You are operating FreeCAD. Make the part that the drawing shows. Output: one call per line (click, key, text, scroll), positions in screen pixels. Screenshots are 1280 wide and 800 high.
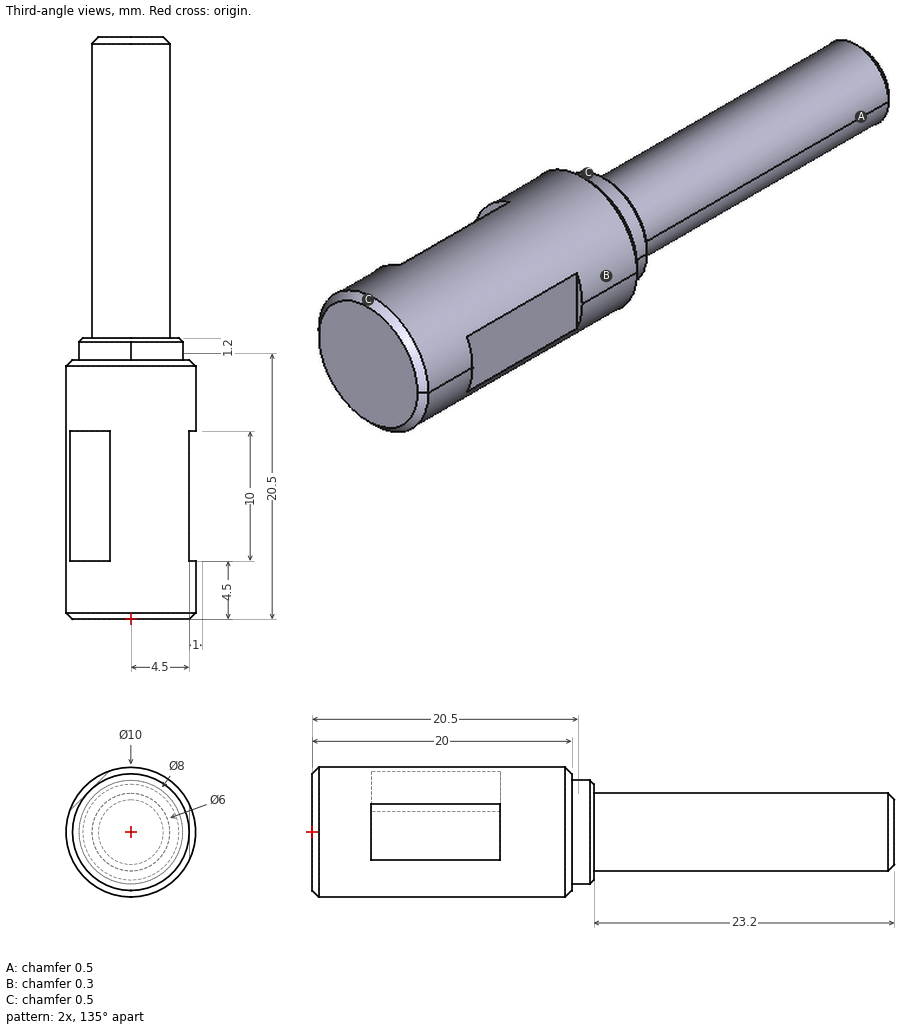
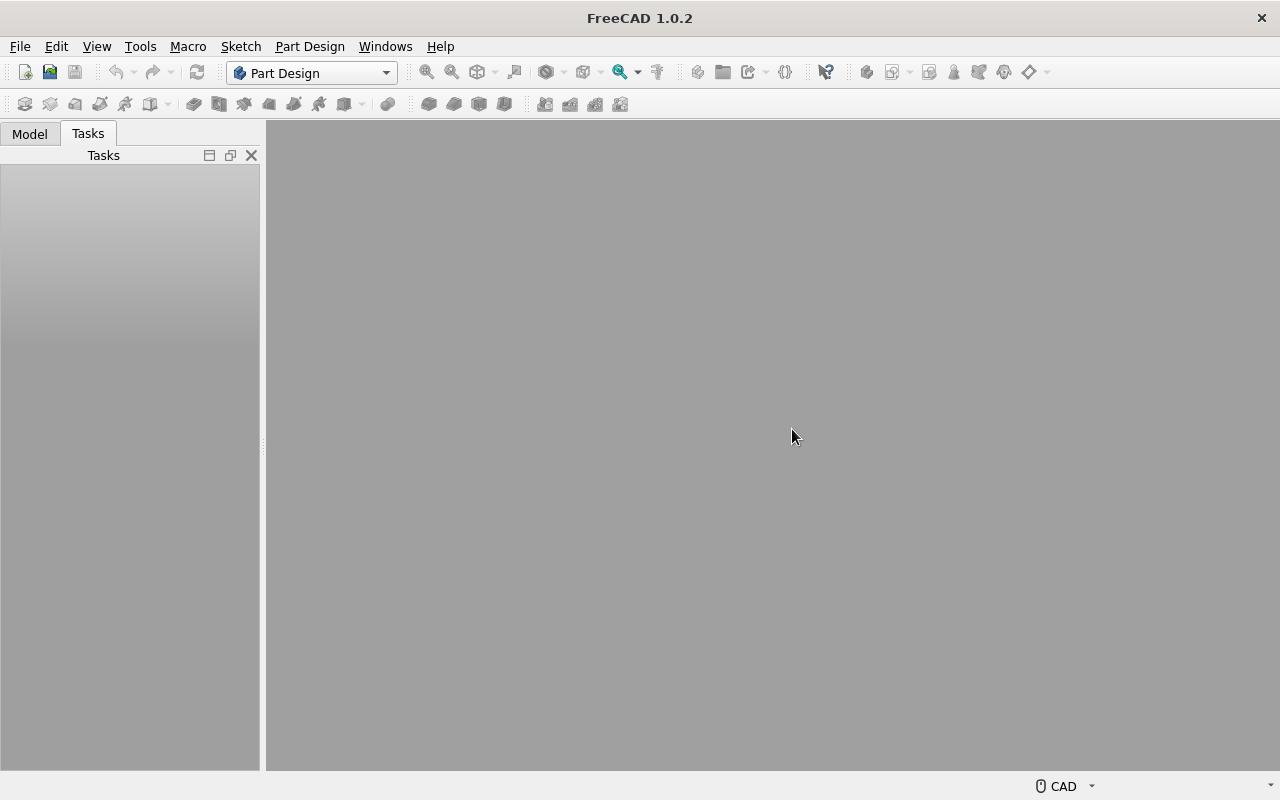
click(25, 72)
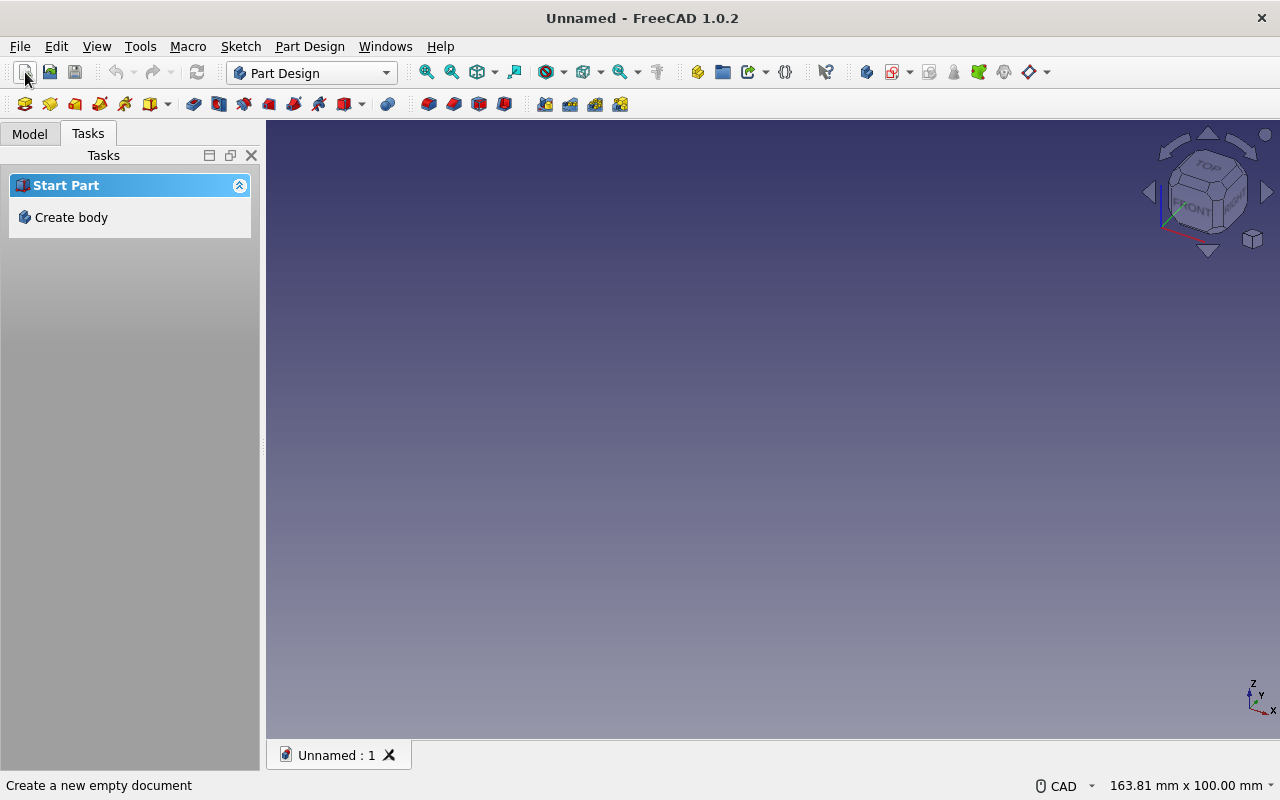
click(892, 72)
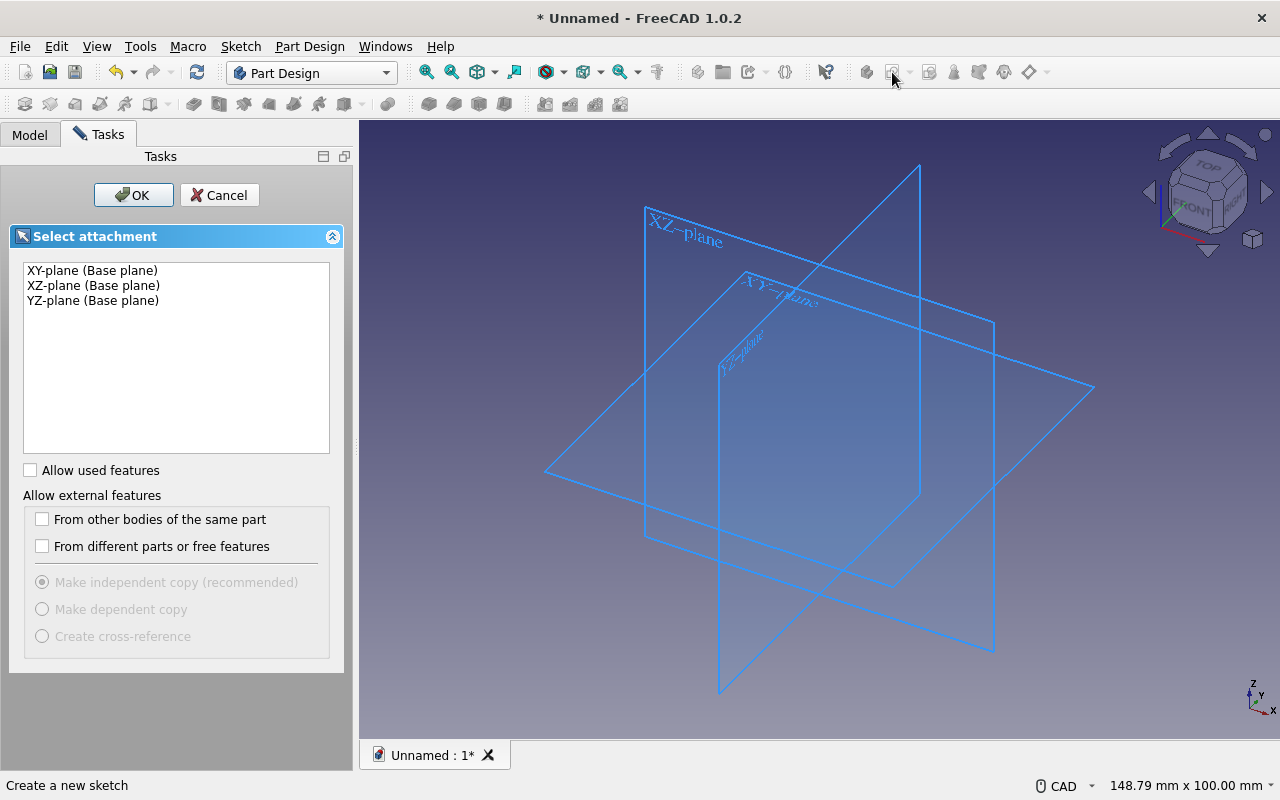
click(84, 286)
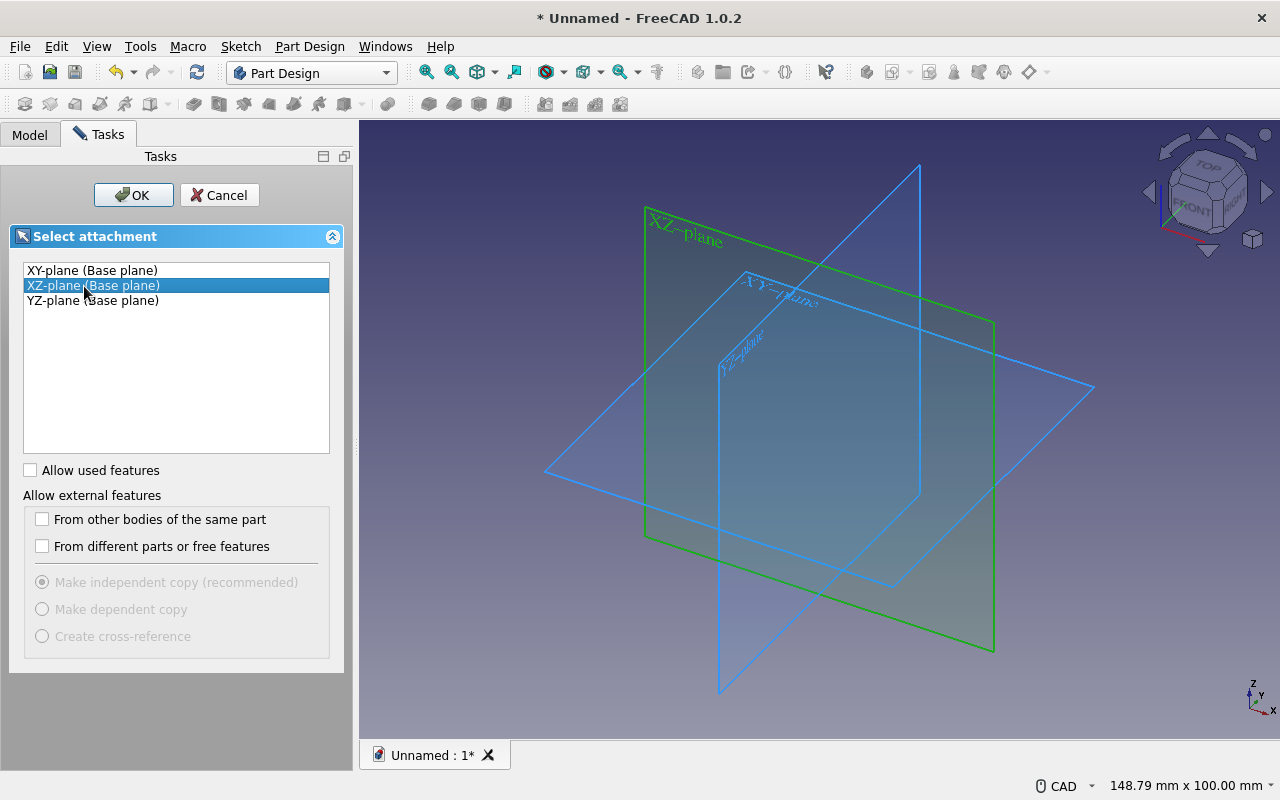
click(134, 195)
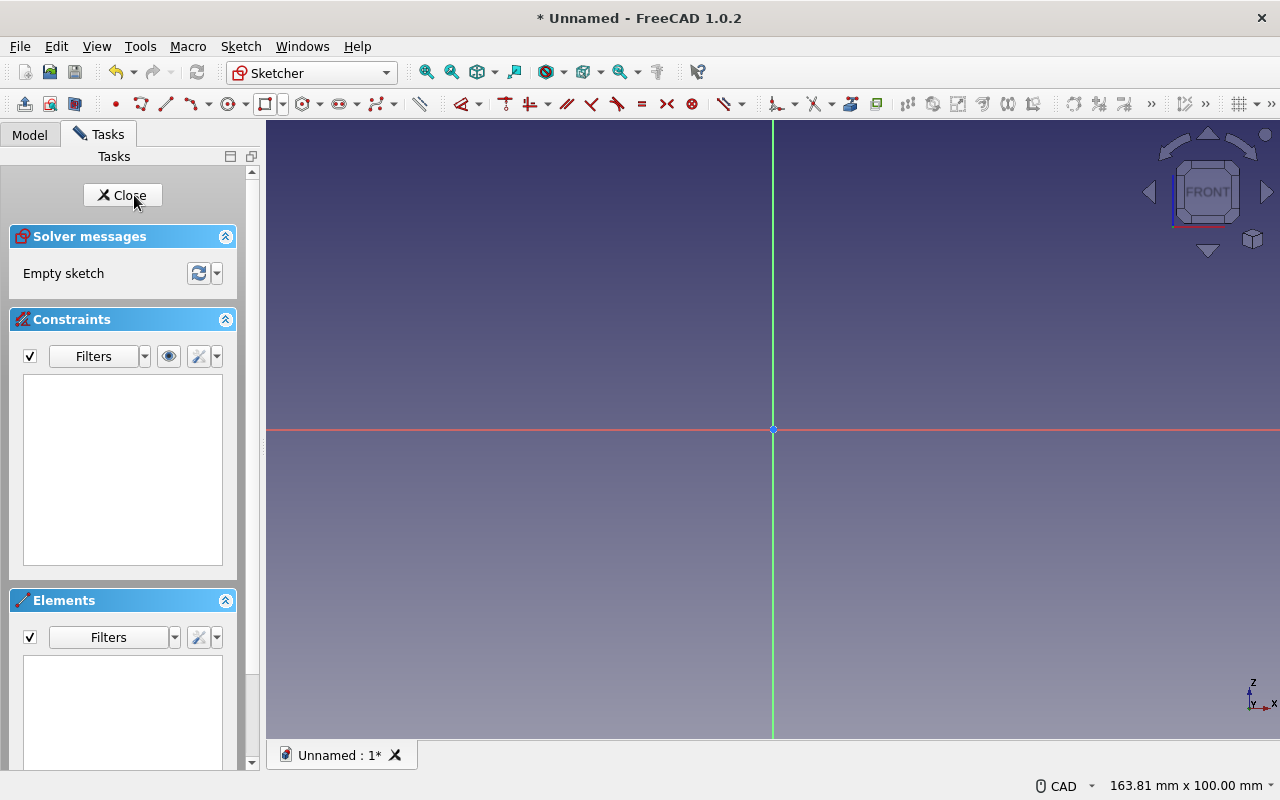
scroll(780, 429, up, 12)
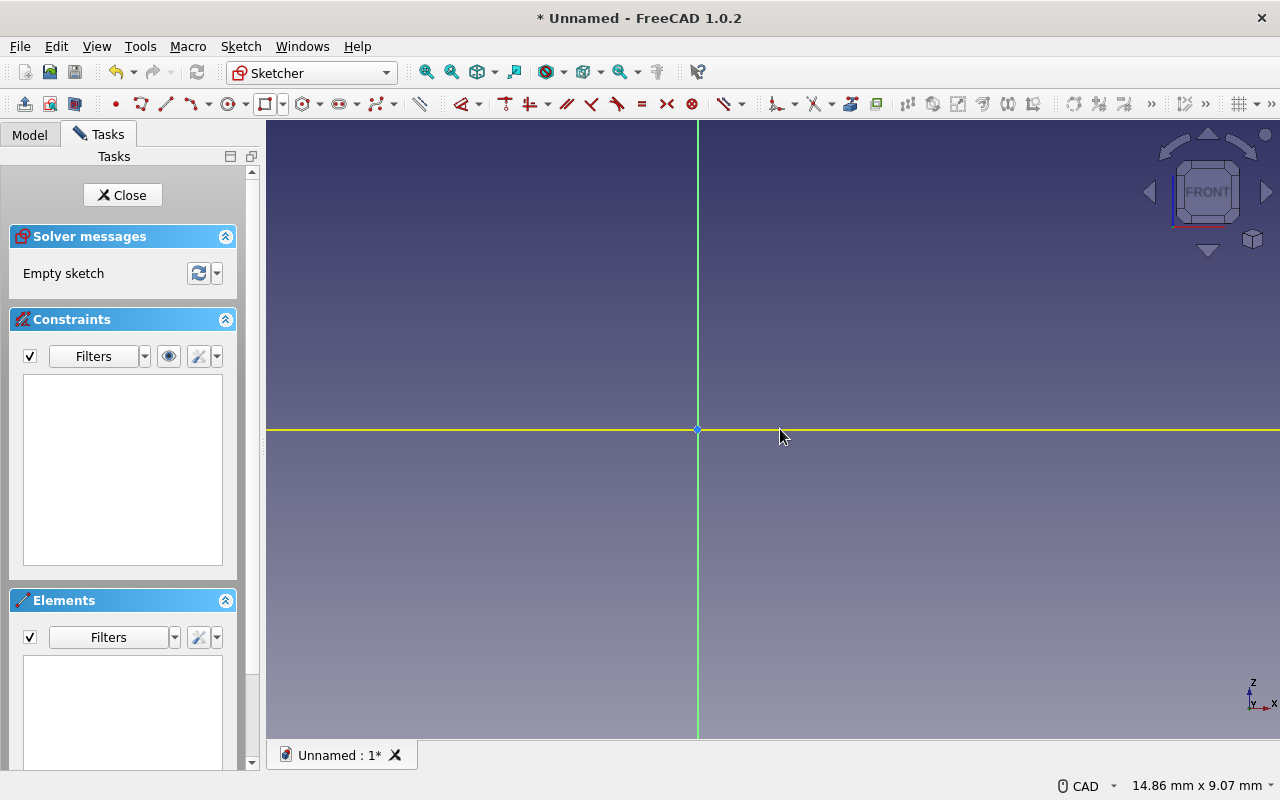
click(228, 104)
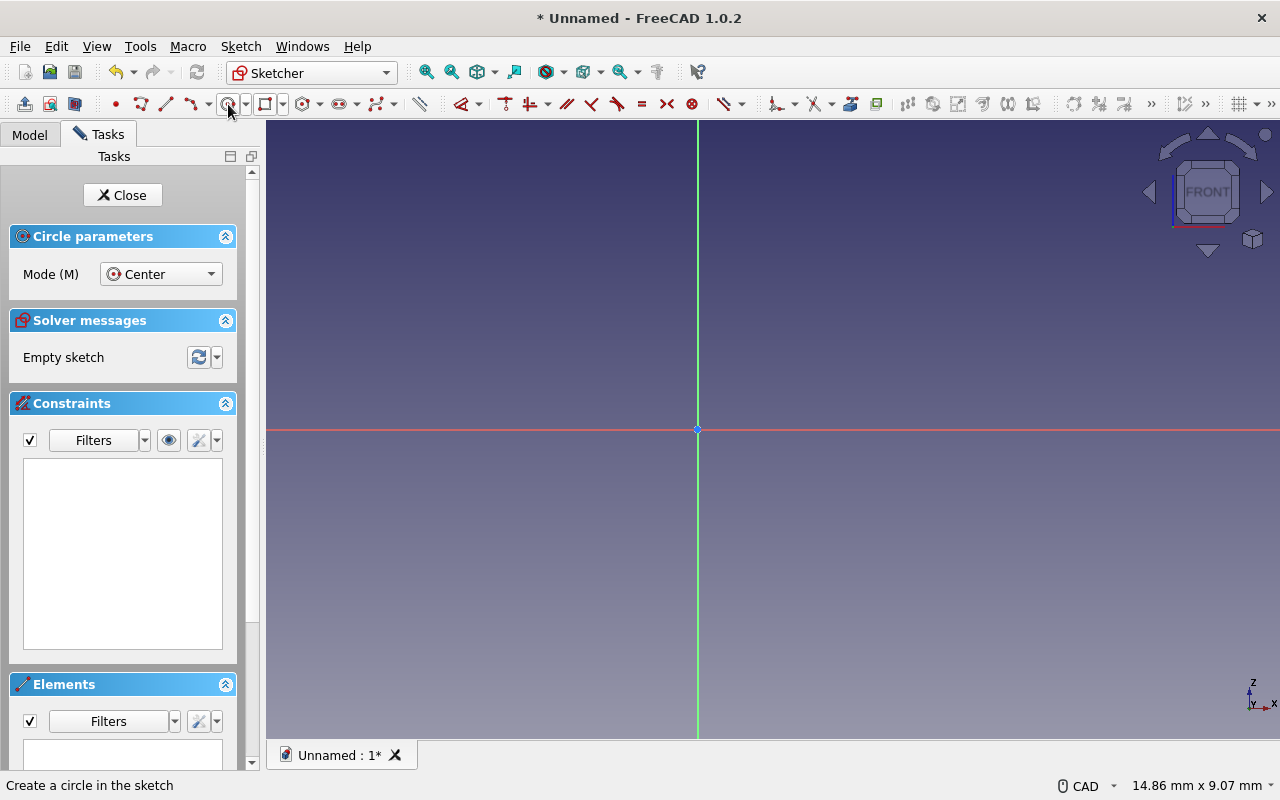
click(698, 430)
move(842, 285)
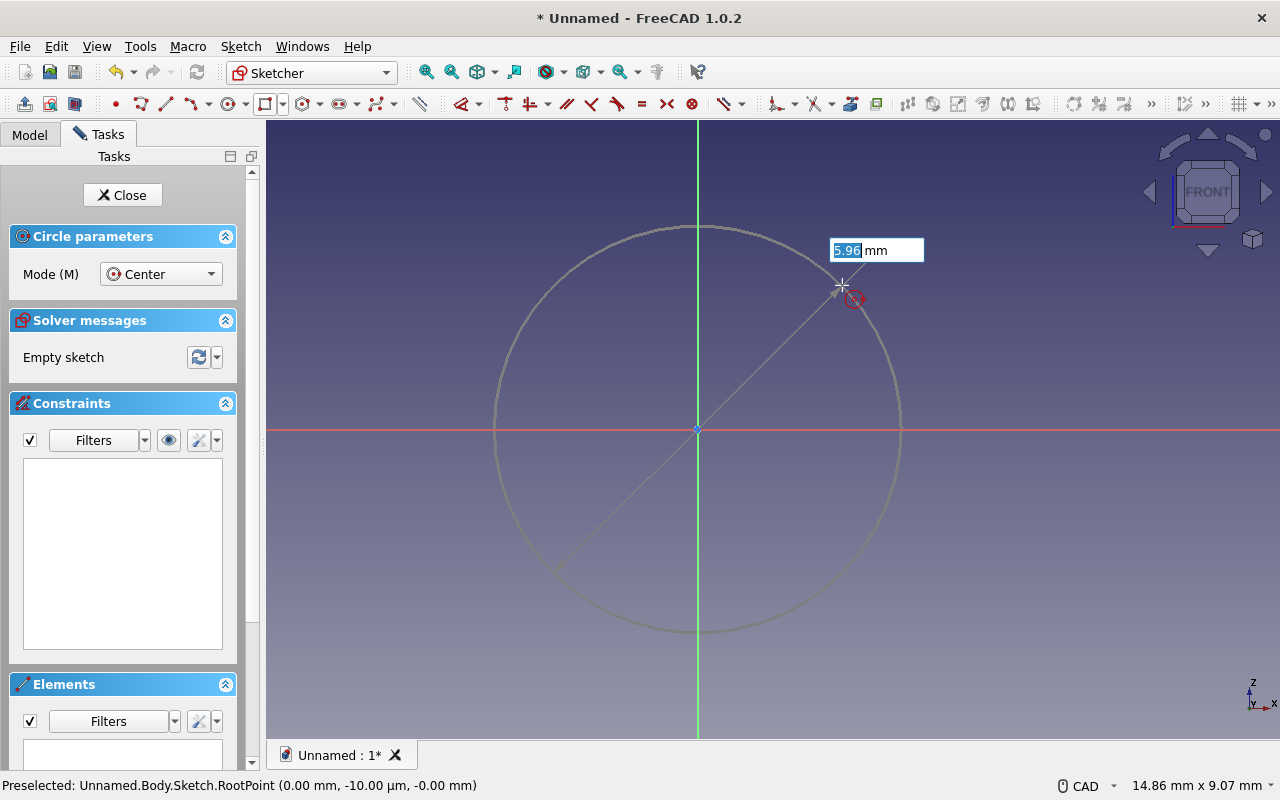
text(6)
key(Return)
key(Escape)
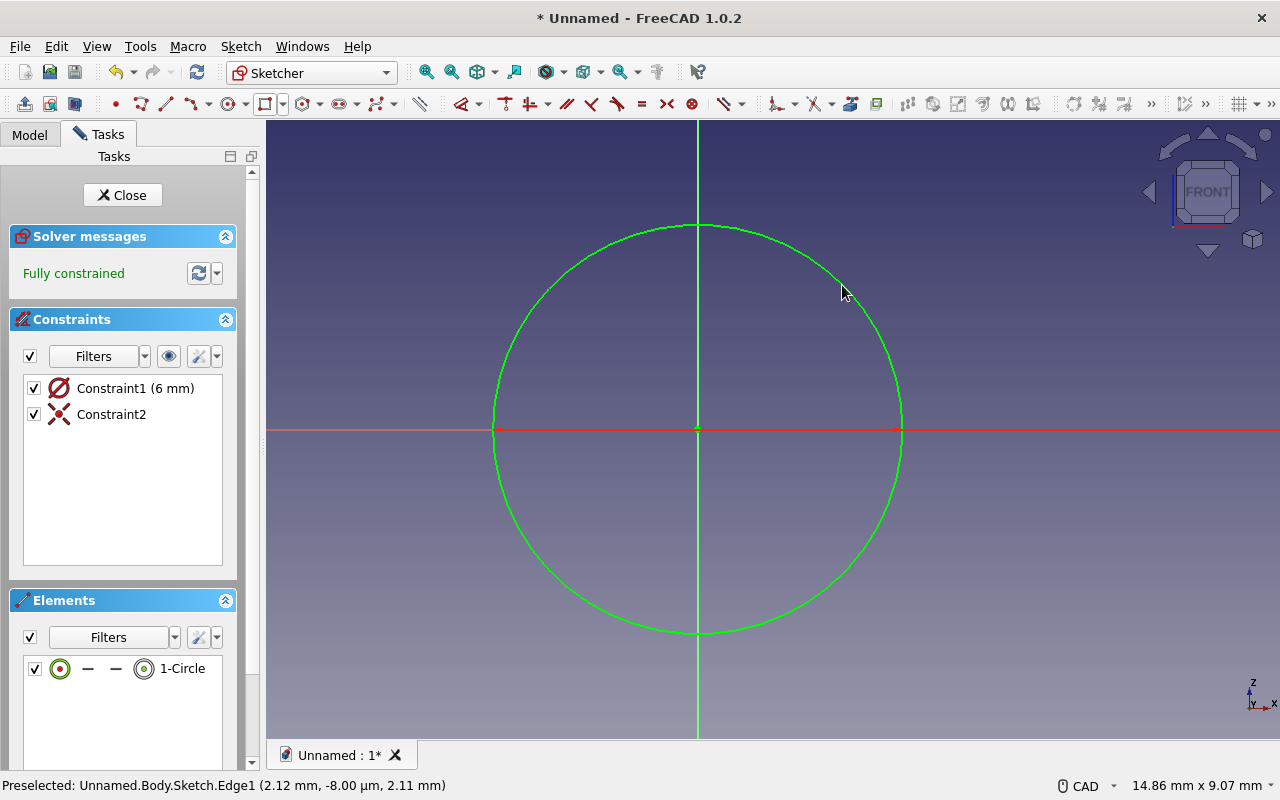
click(123, 195)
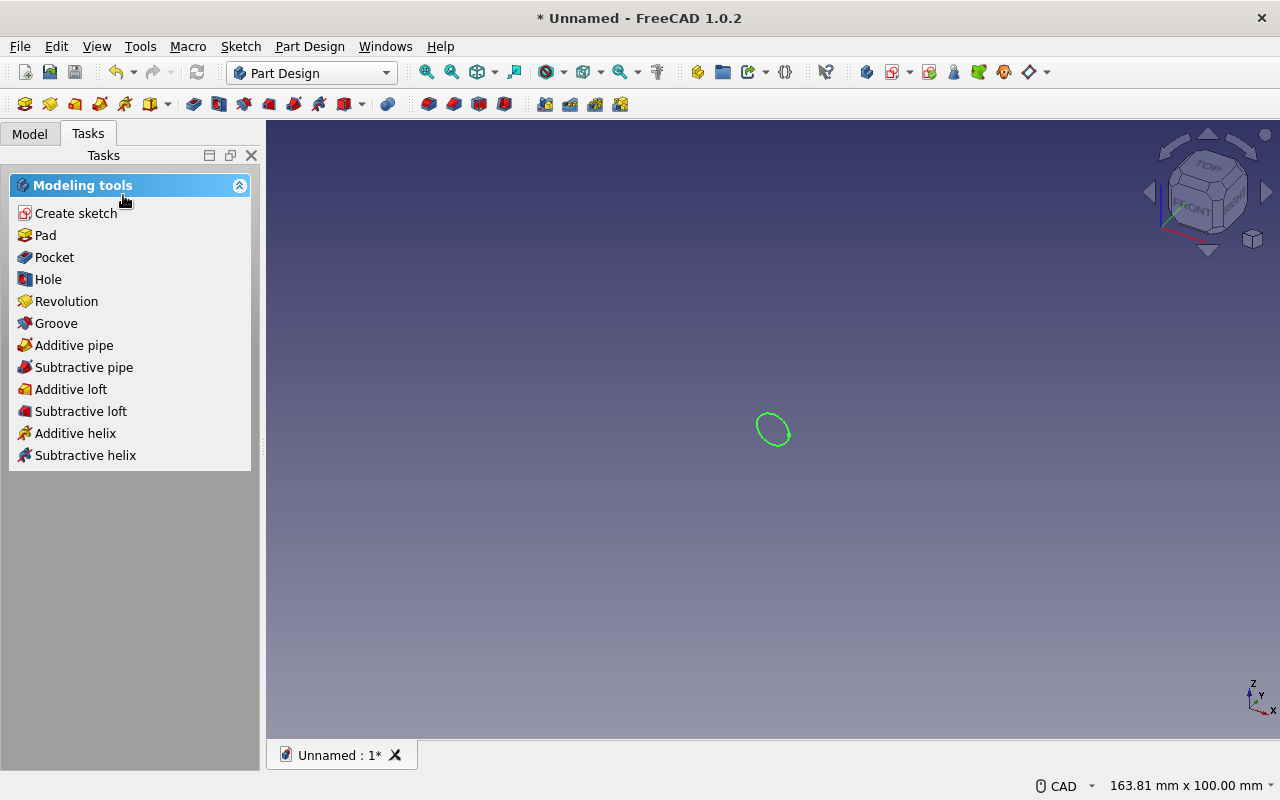
click(25, 104)